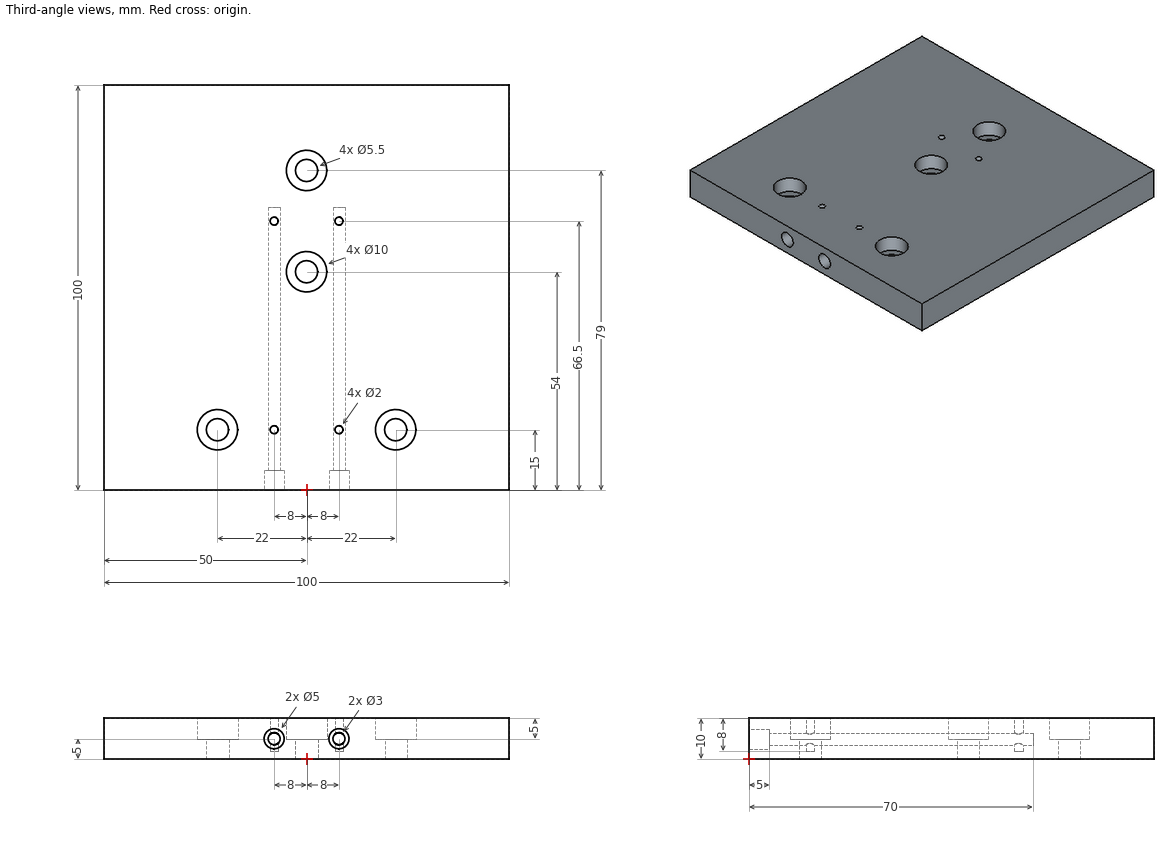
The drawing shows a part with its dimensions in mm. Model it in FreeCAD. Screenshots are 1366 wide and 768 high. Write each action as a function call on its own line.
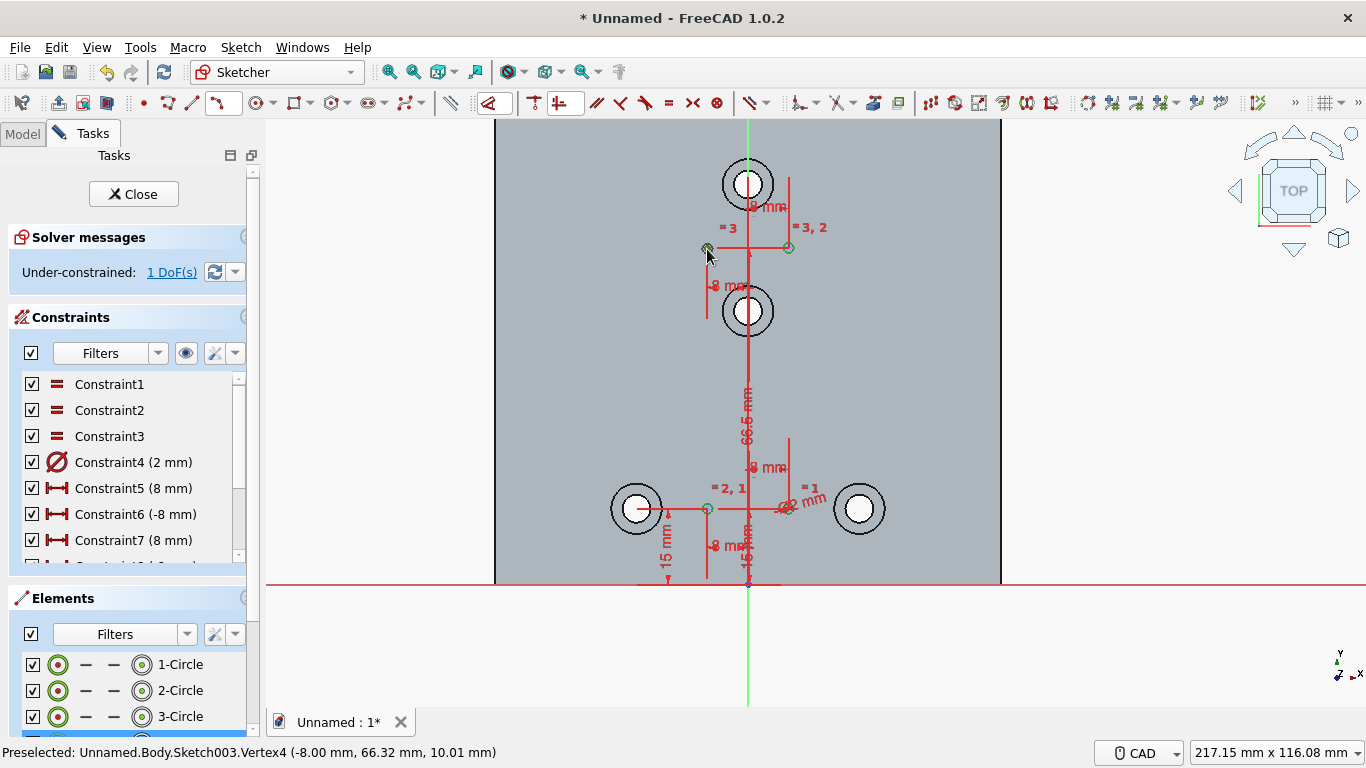
click(506, 104)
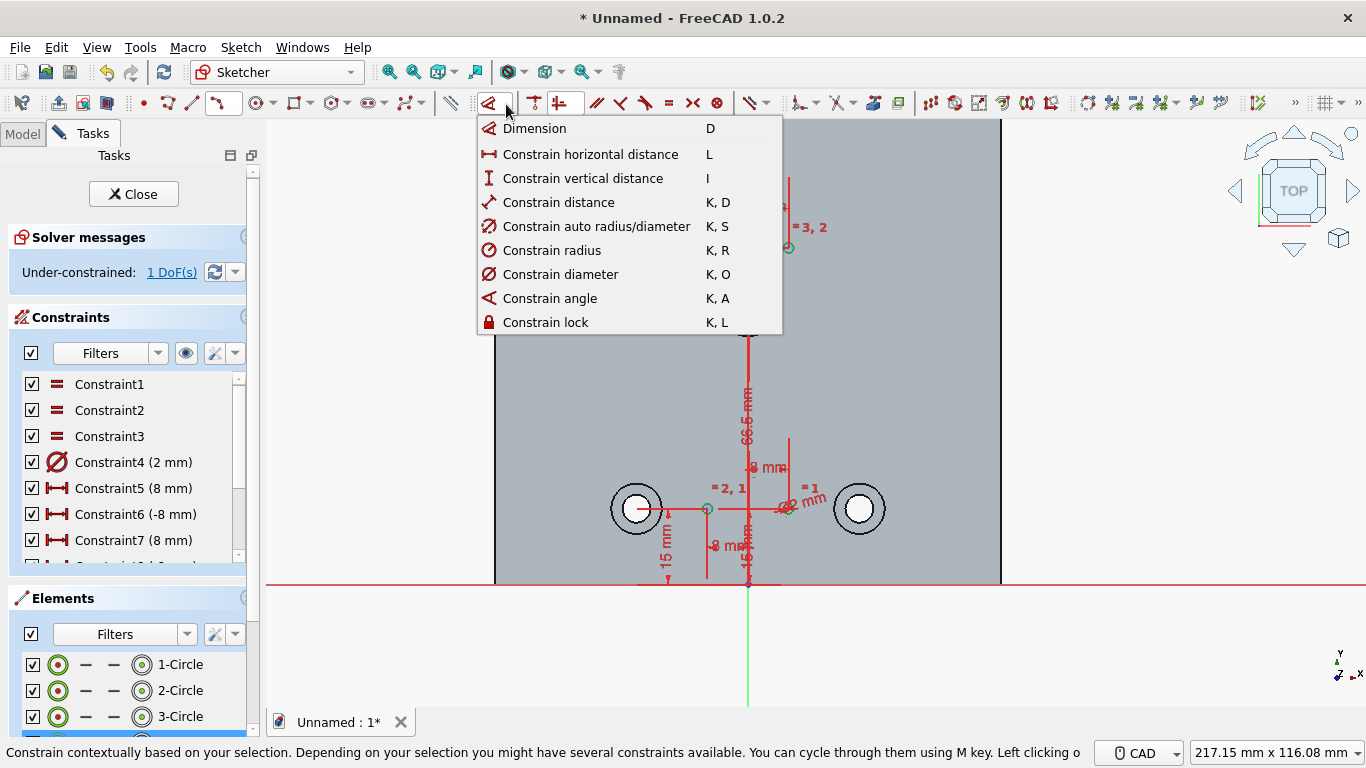
click(630, 178)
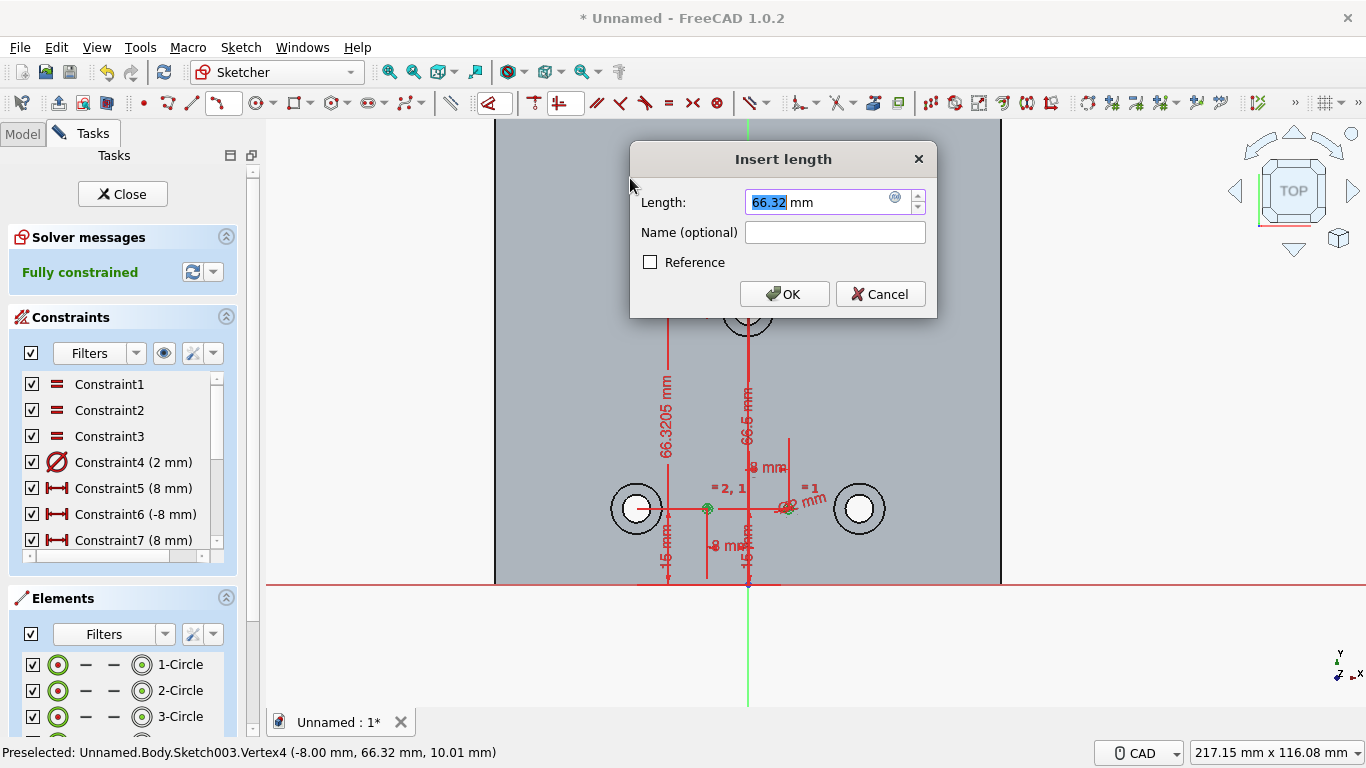
text(66.5)
key(Return)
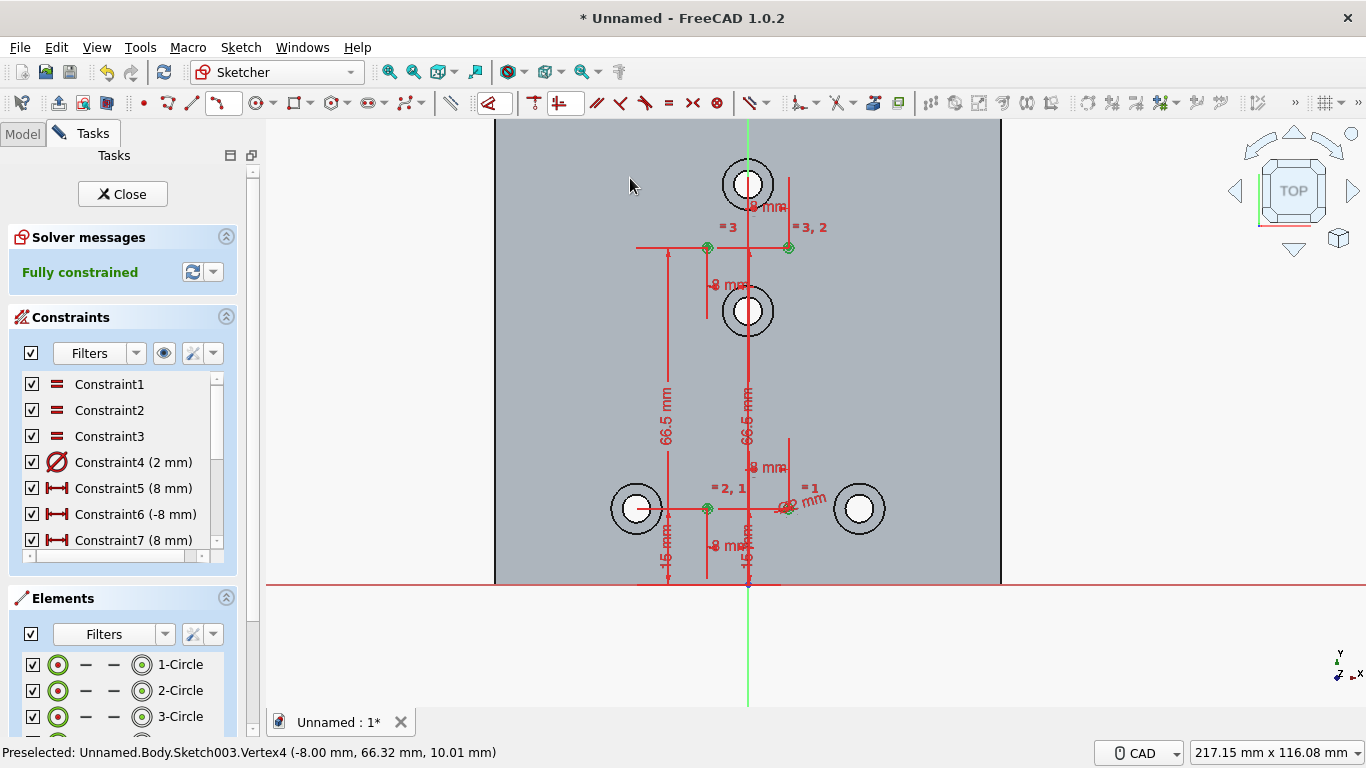
click(123, 194)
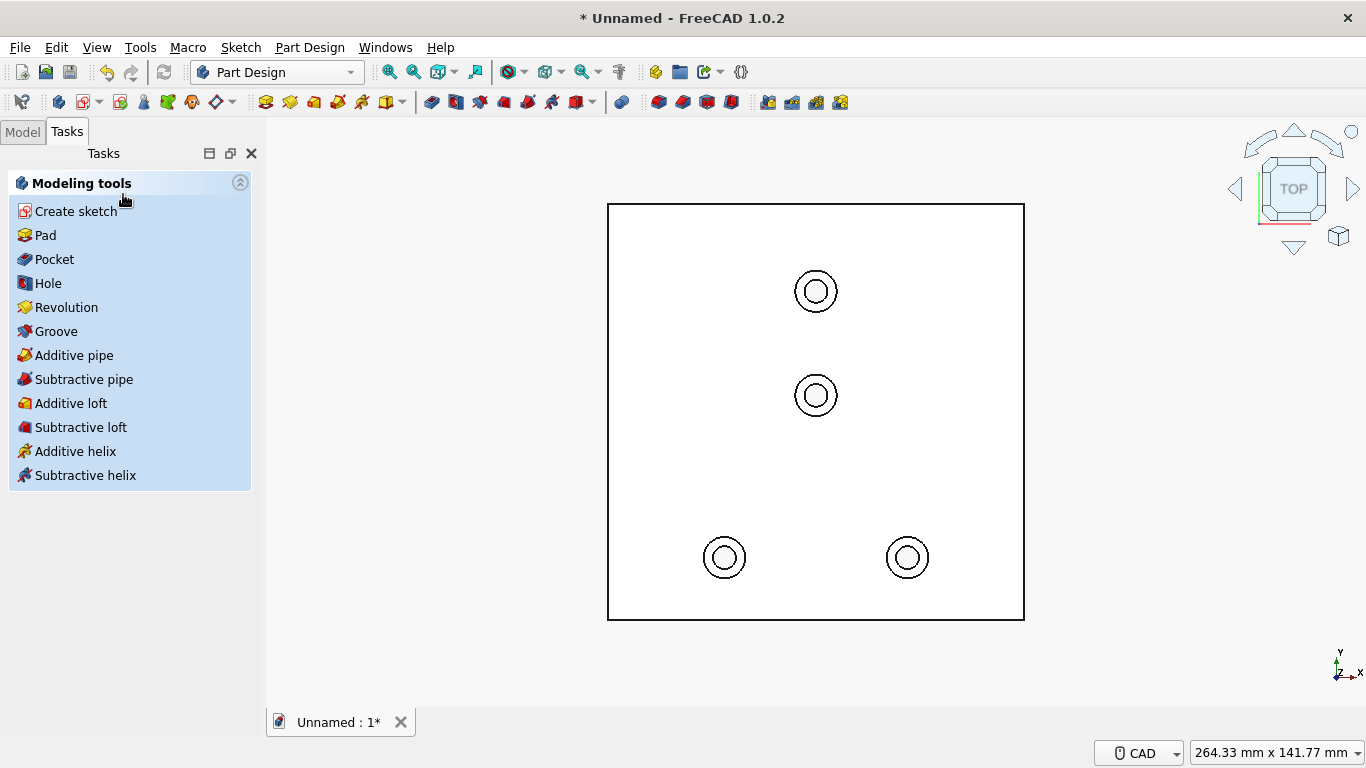
click(432, 102)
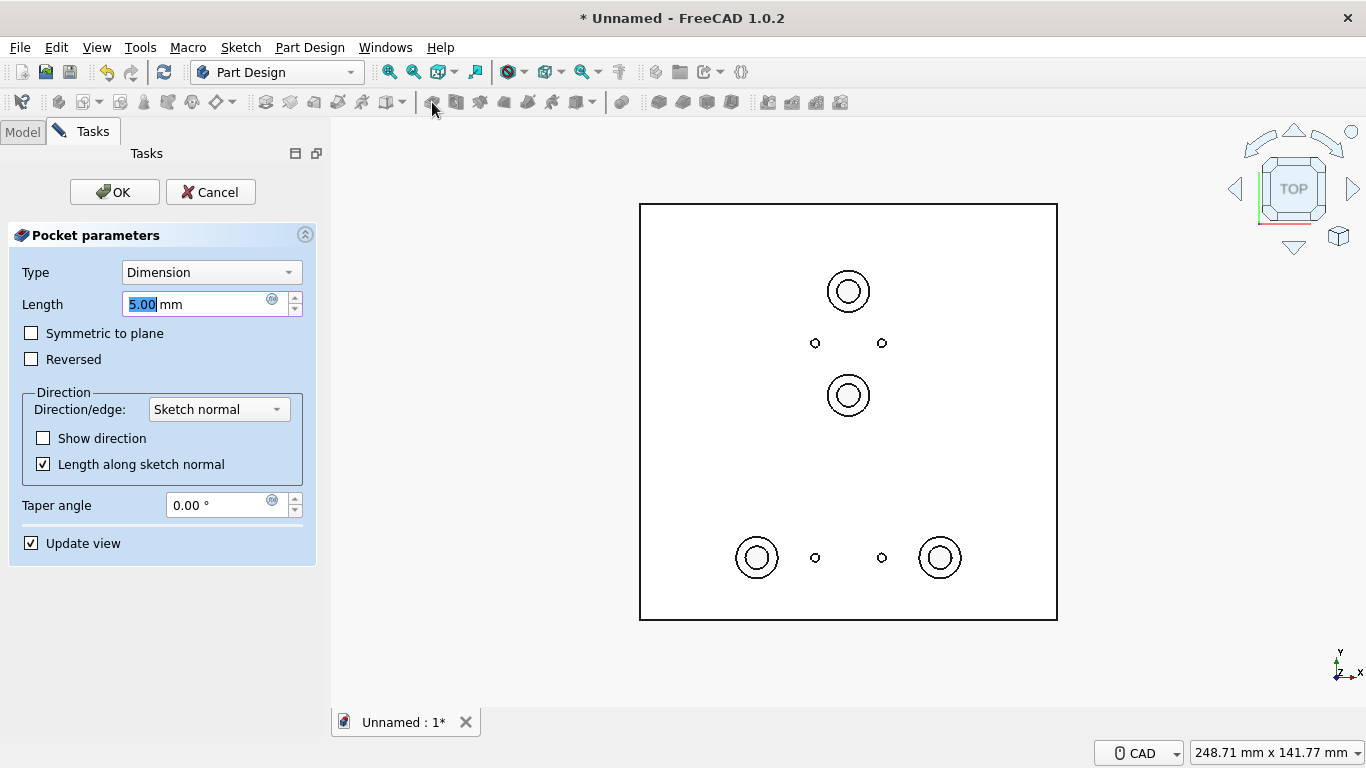
text(8)
key(Tab)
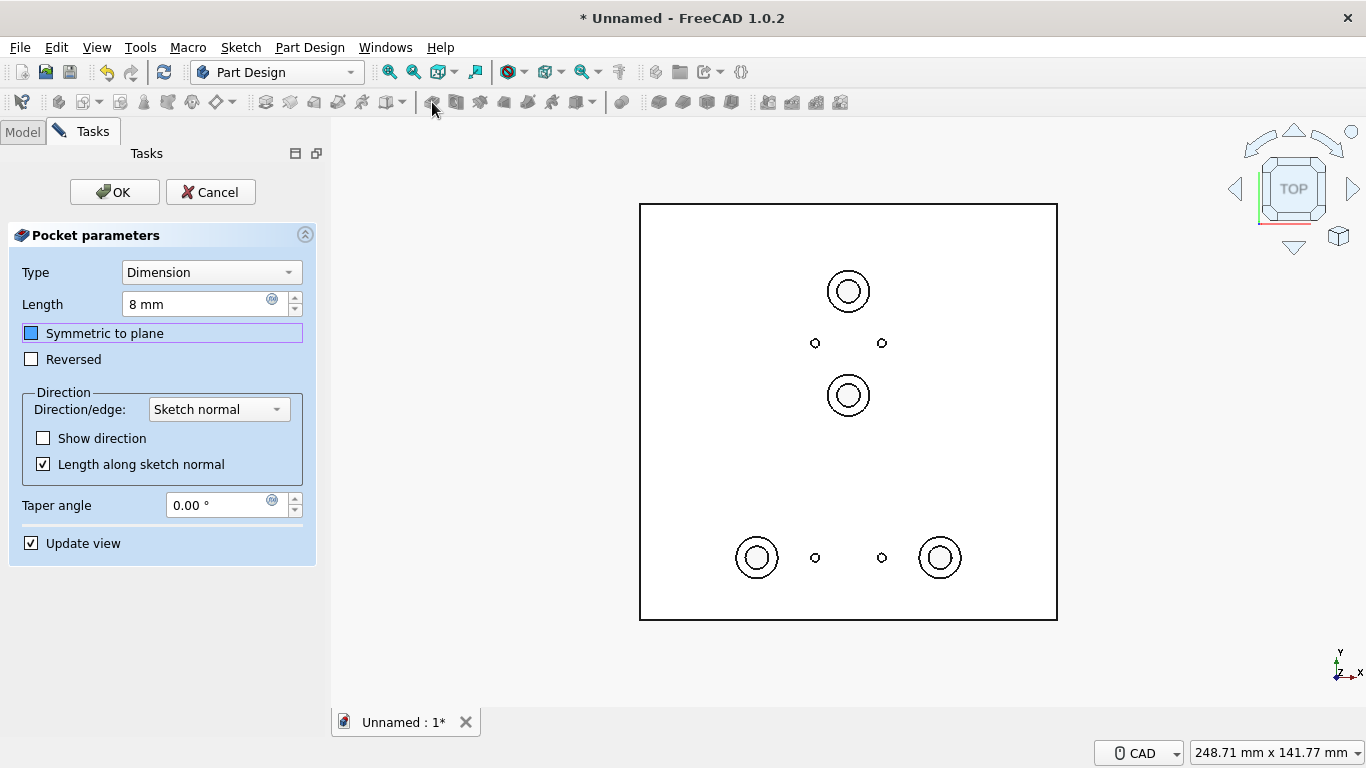
click(115, 192)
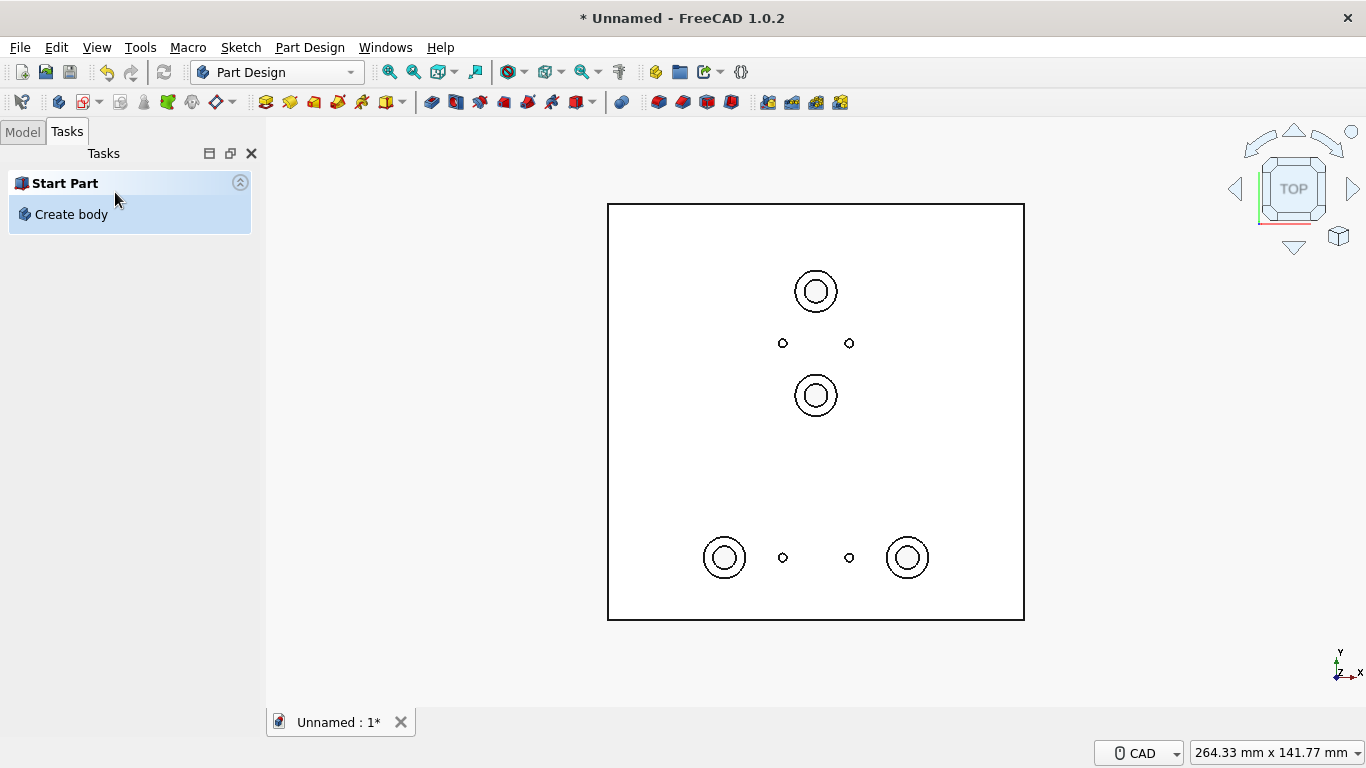
click(84, 102)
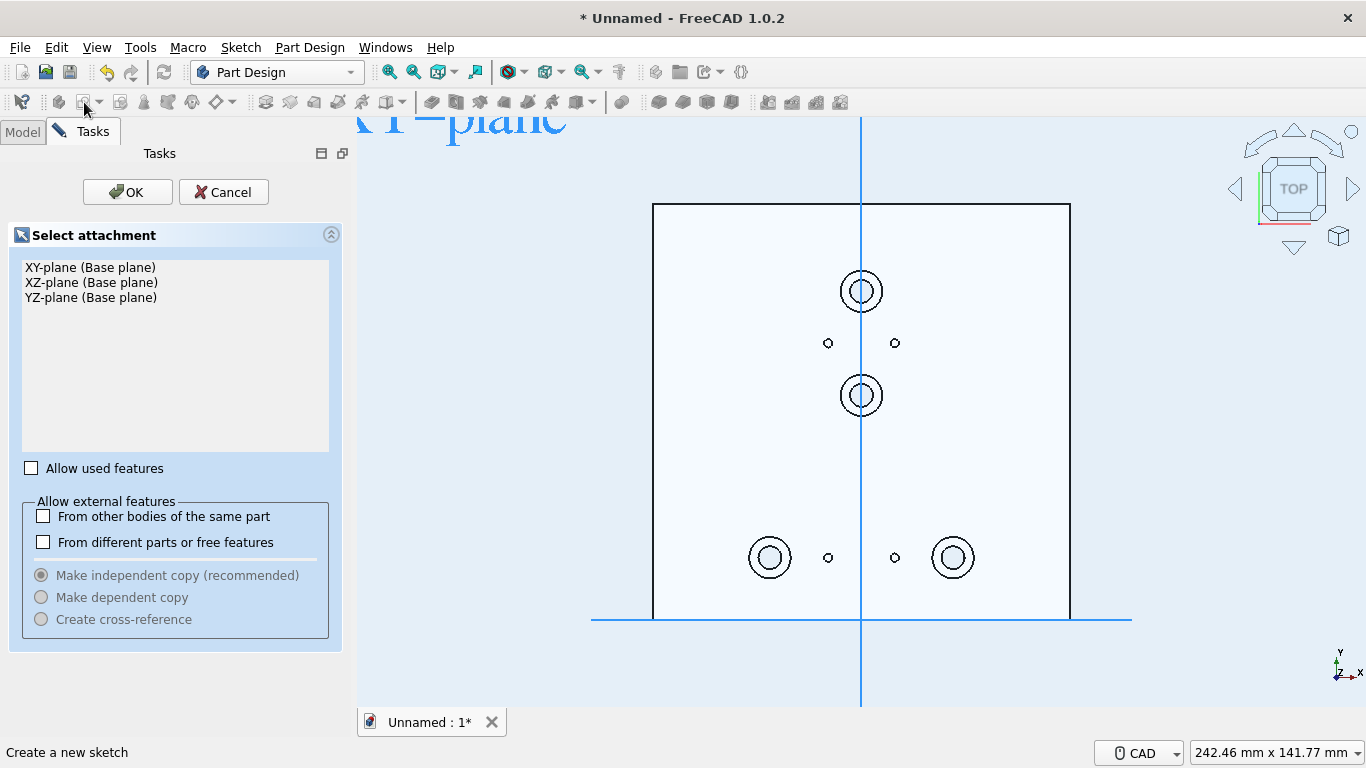
click(82, 282)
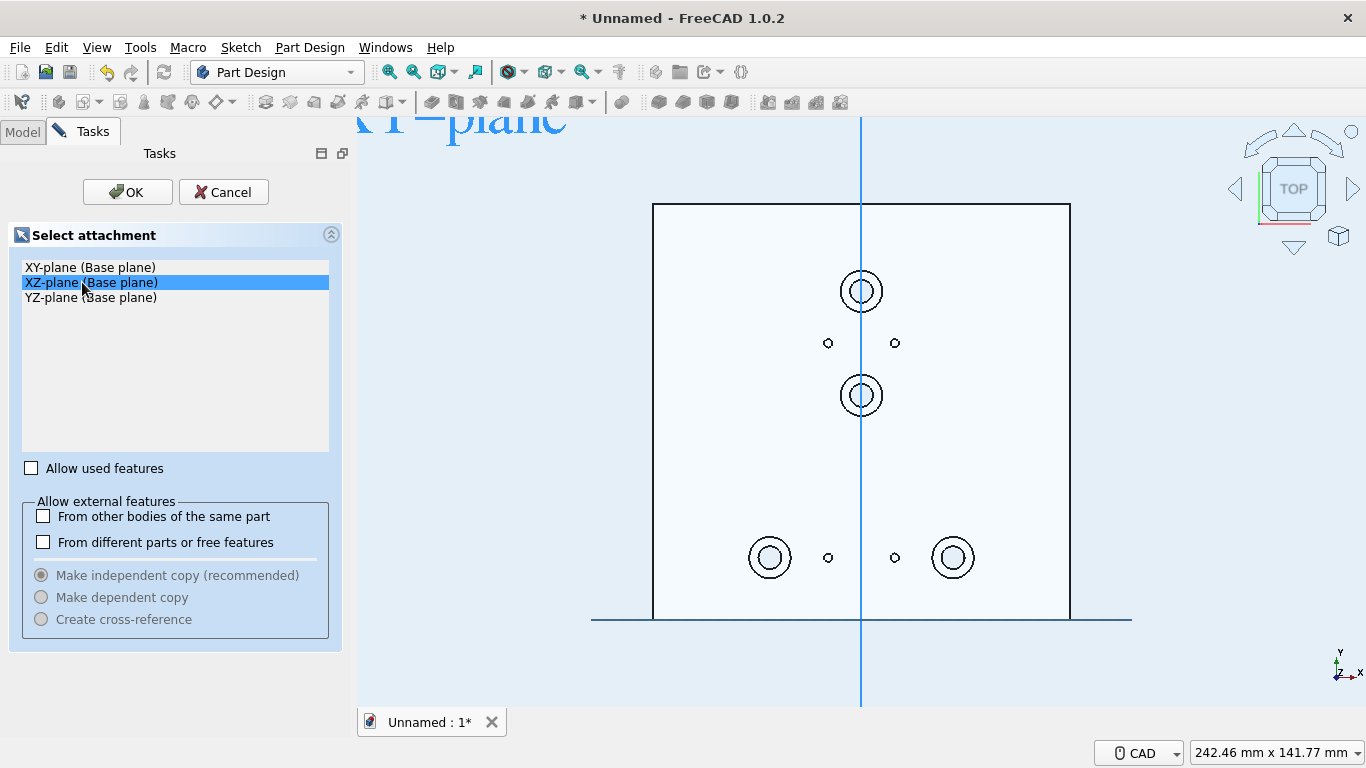
click(128, 192)